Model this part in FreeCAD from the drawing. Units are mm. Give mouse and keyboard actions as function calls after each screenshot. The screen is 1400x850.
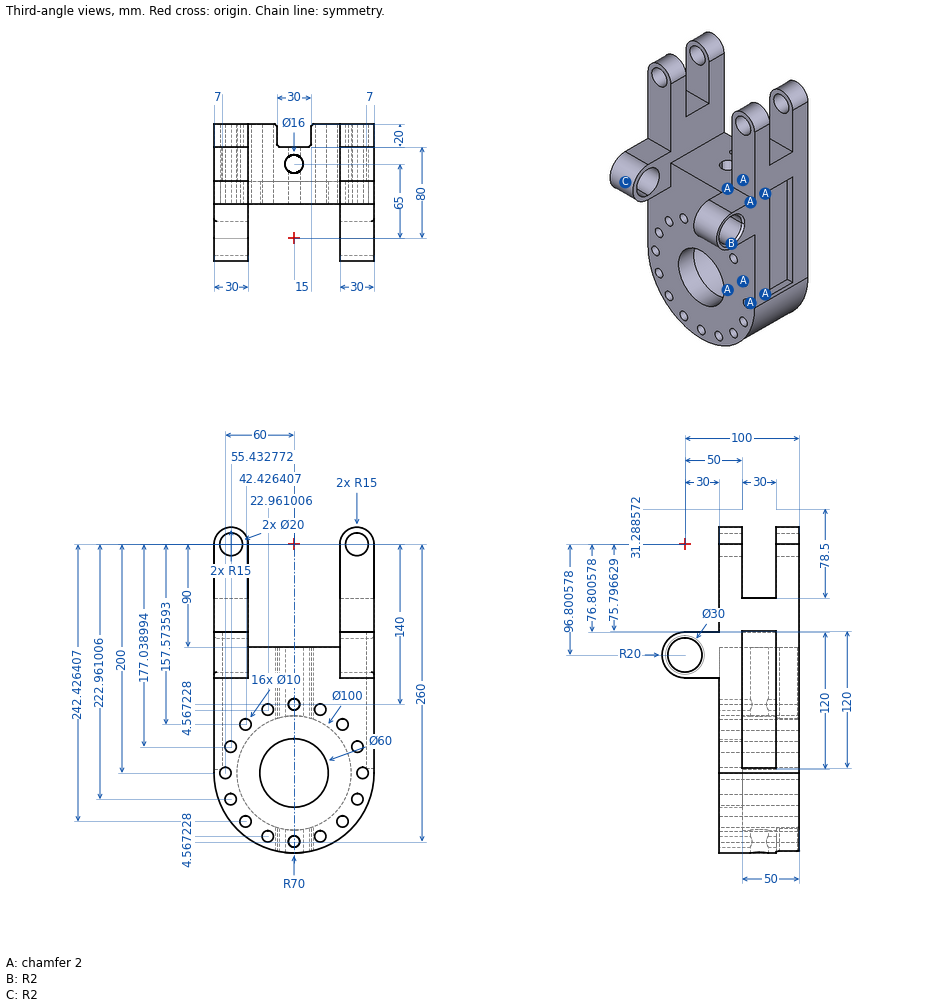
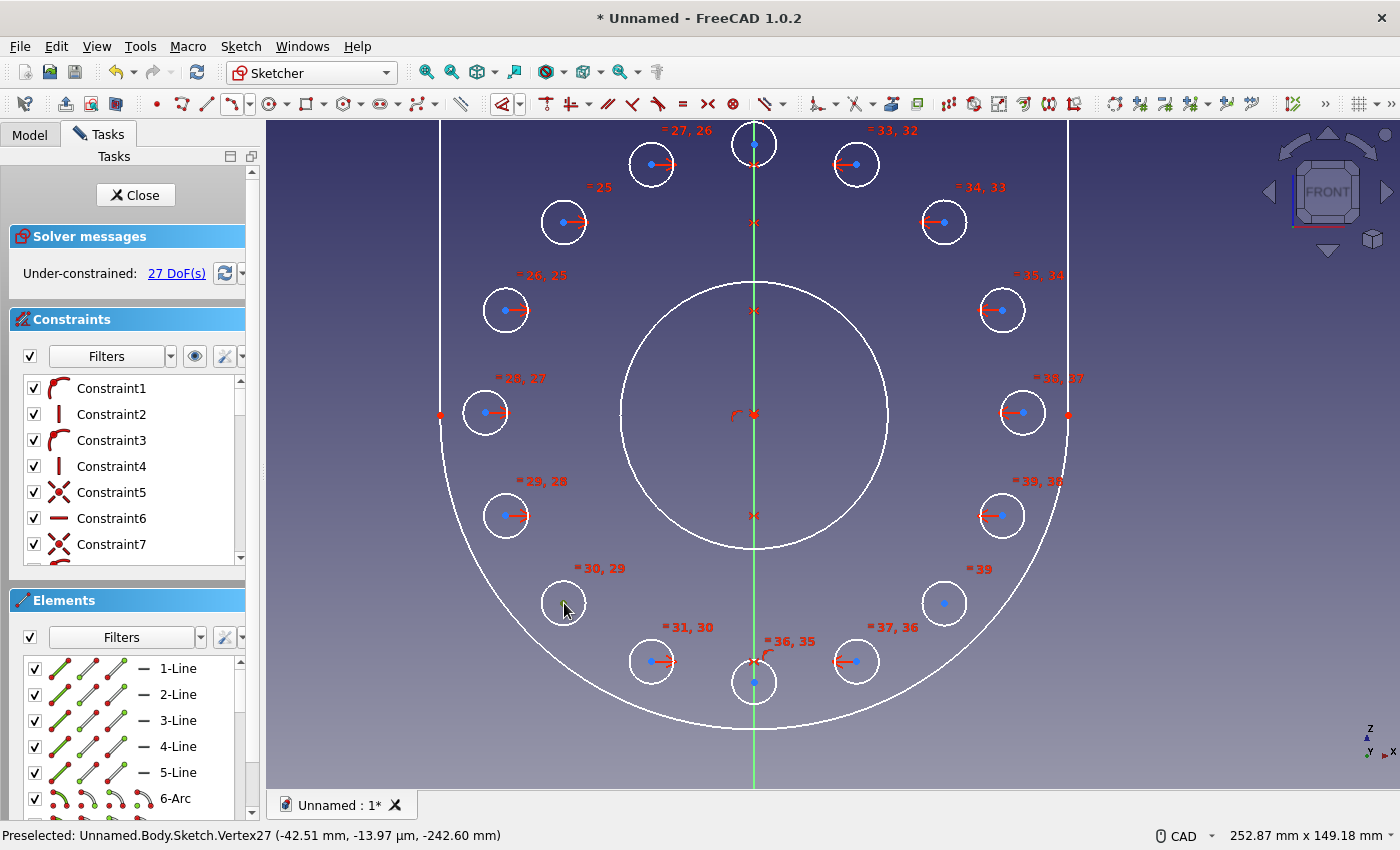
click(944, 604)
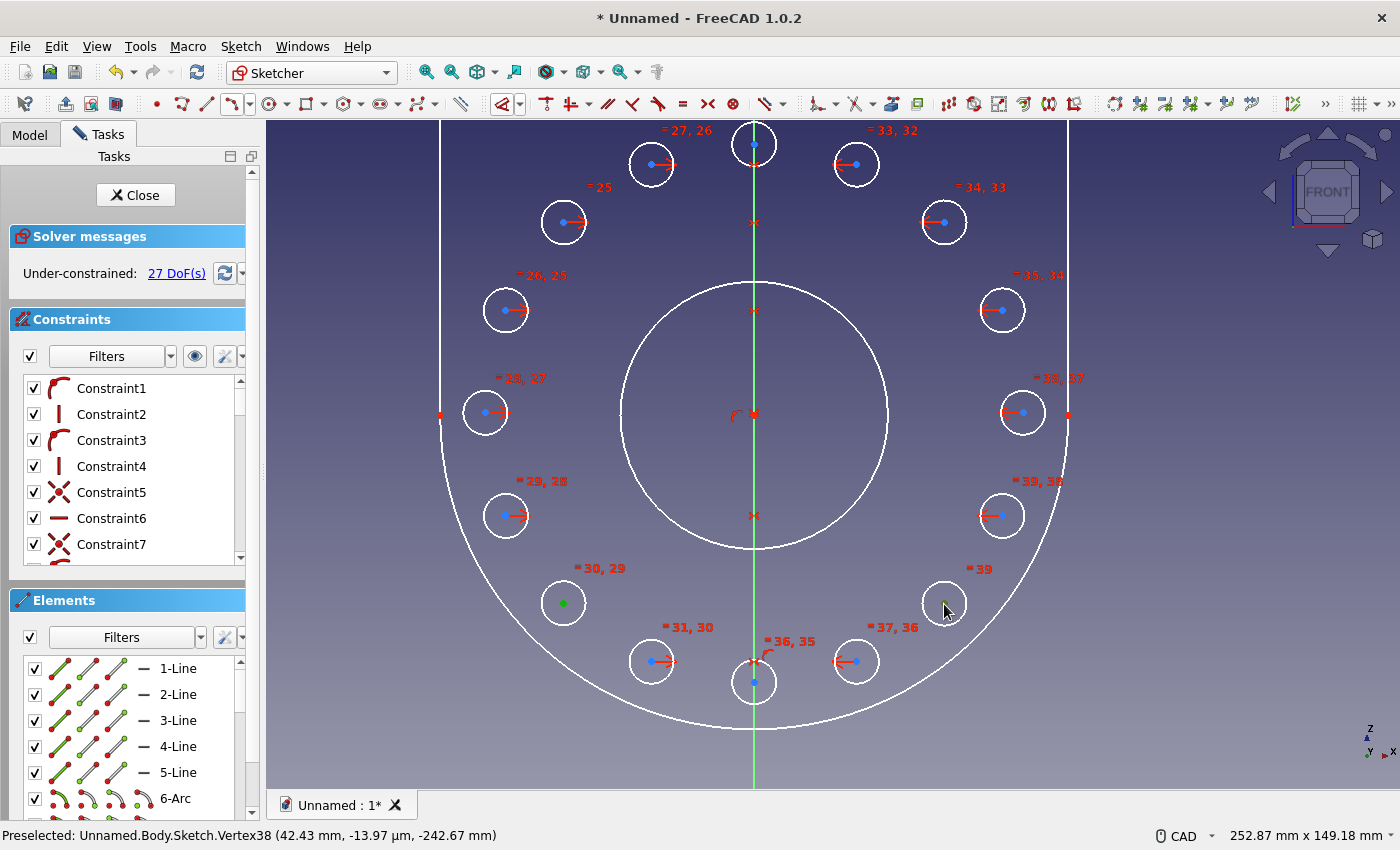
click(754, 630)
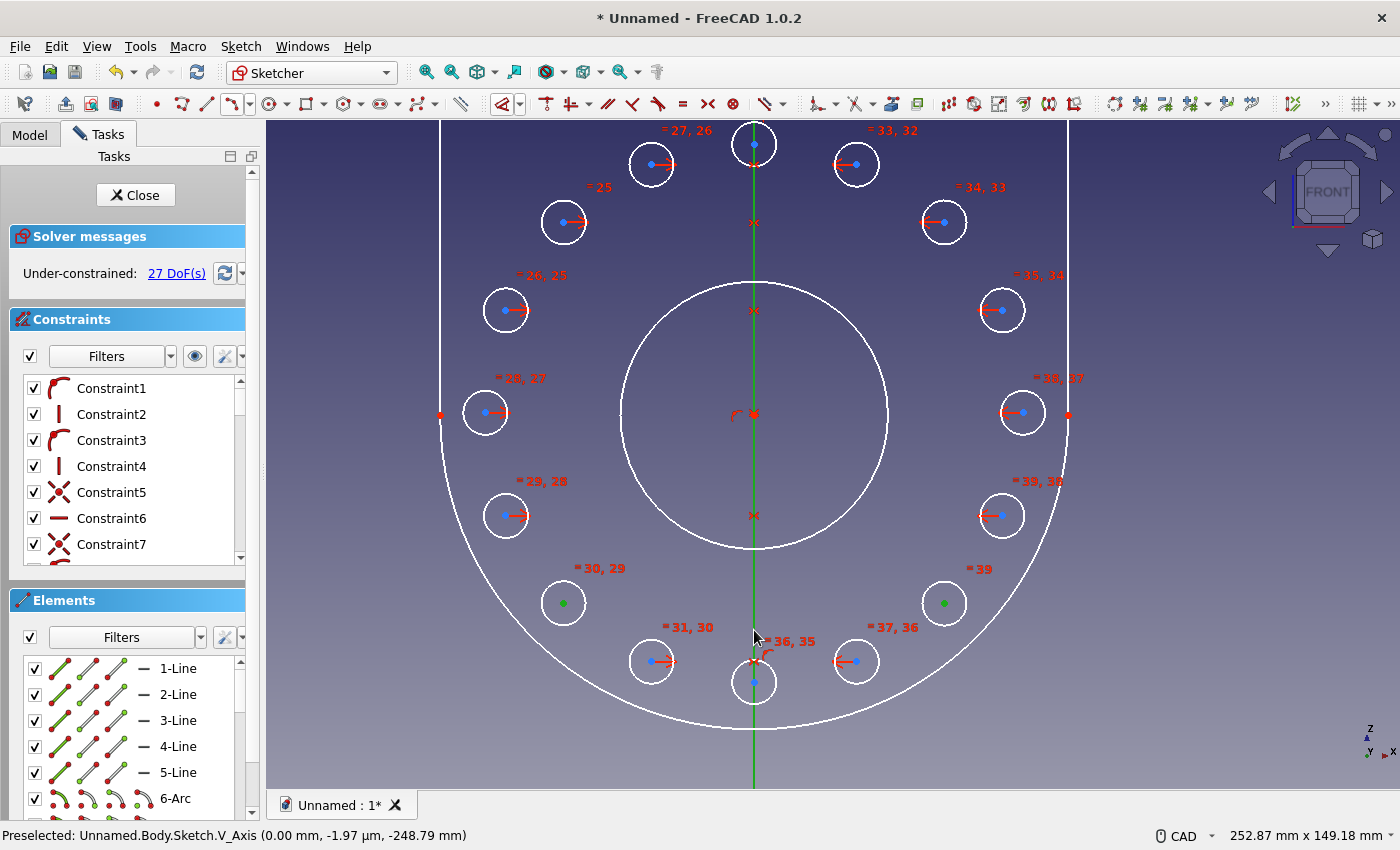
click(708, 104)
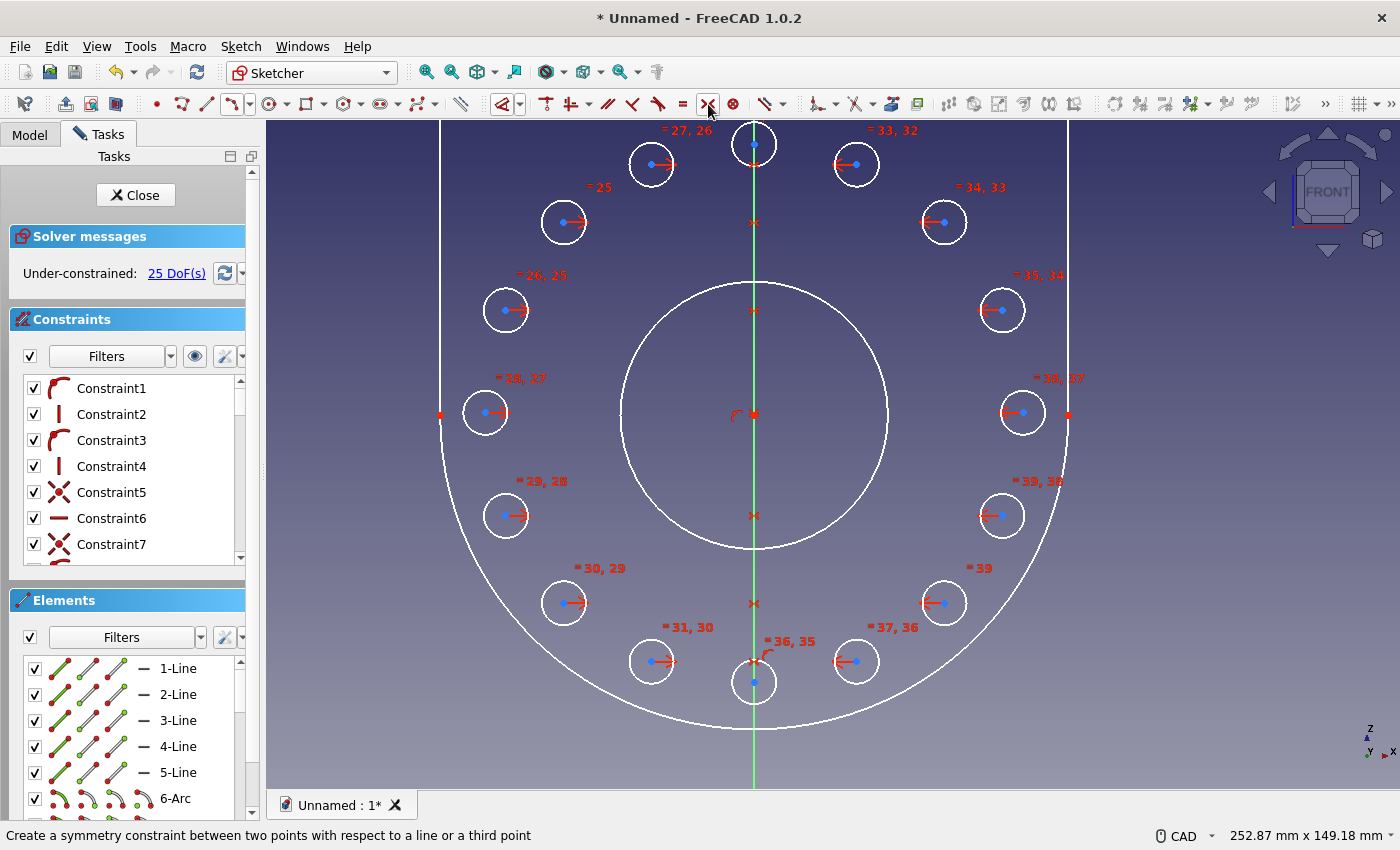
key(d)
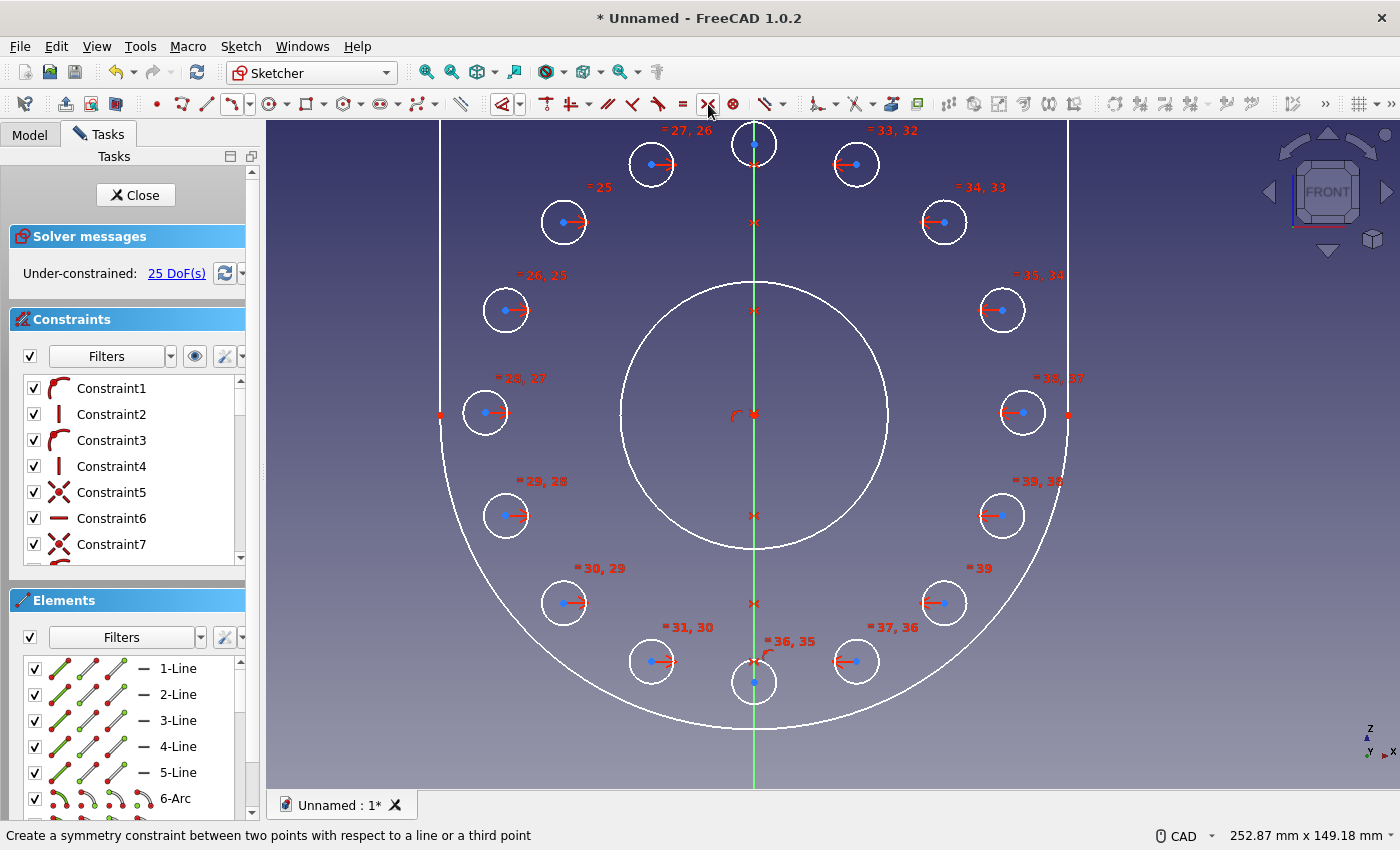
scroll(770, 668, down, 5)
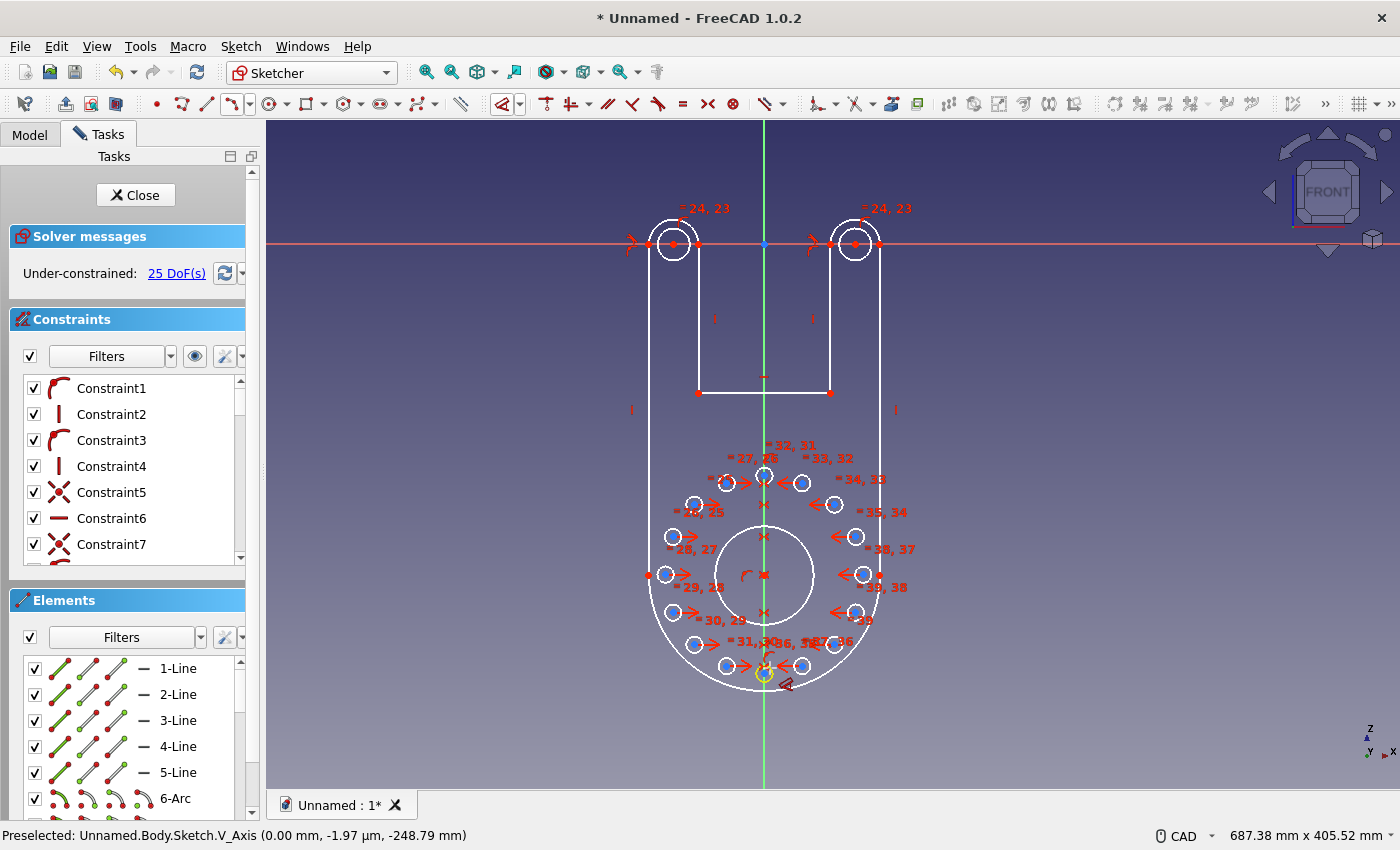
scroll(688, 224, up, 3)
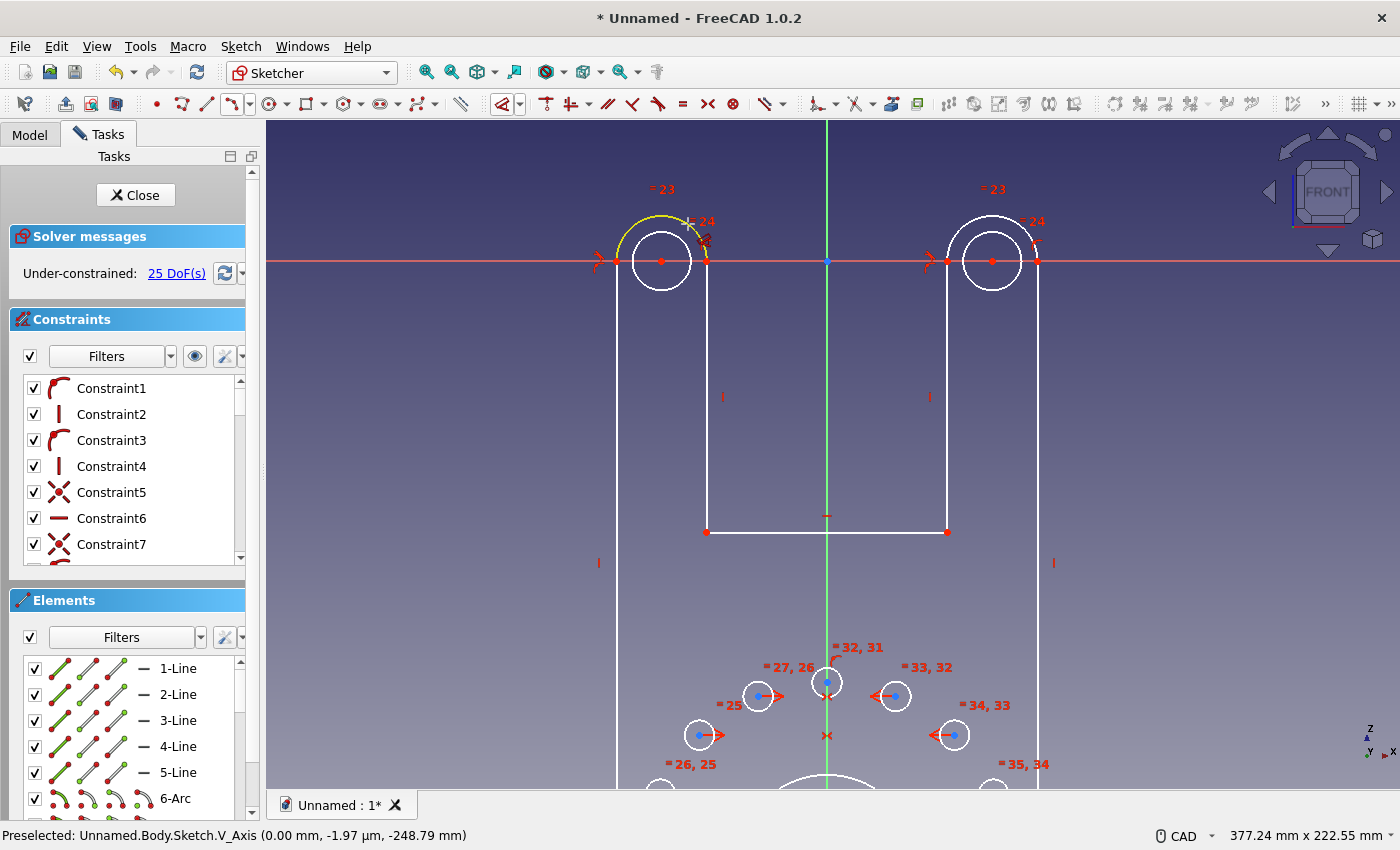
click(688, 225)
click(707, 199)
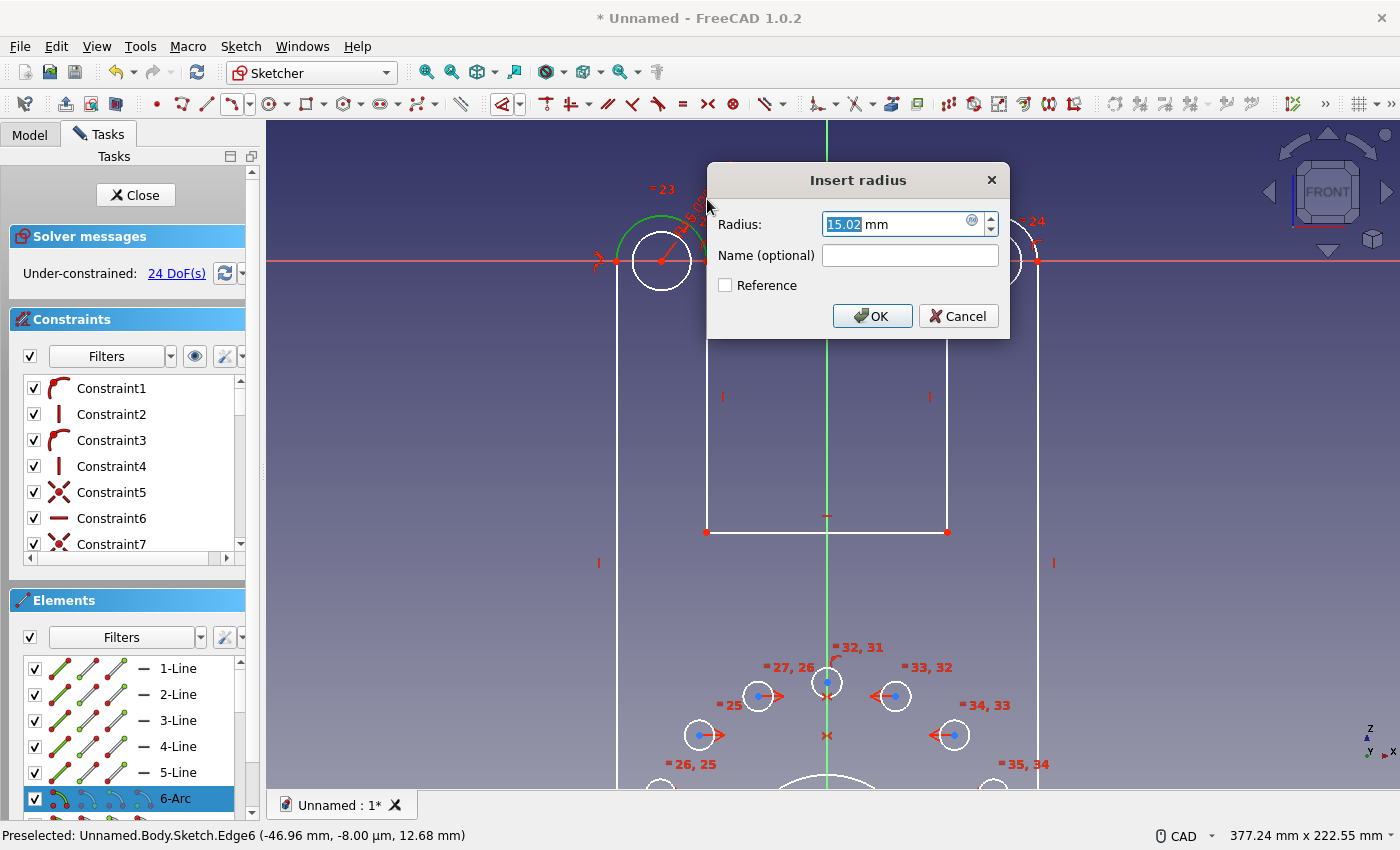
text(15)
key(Return)